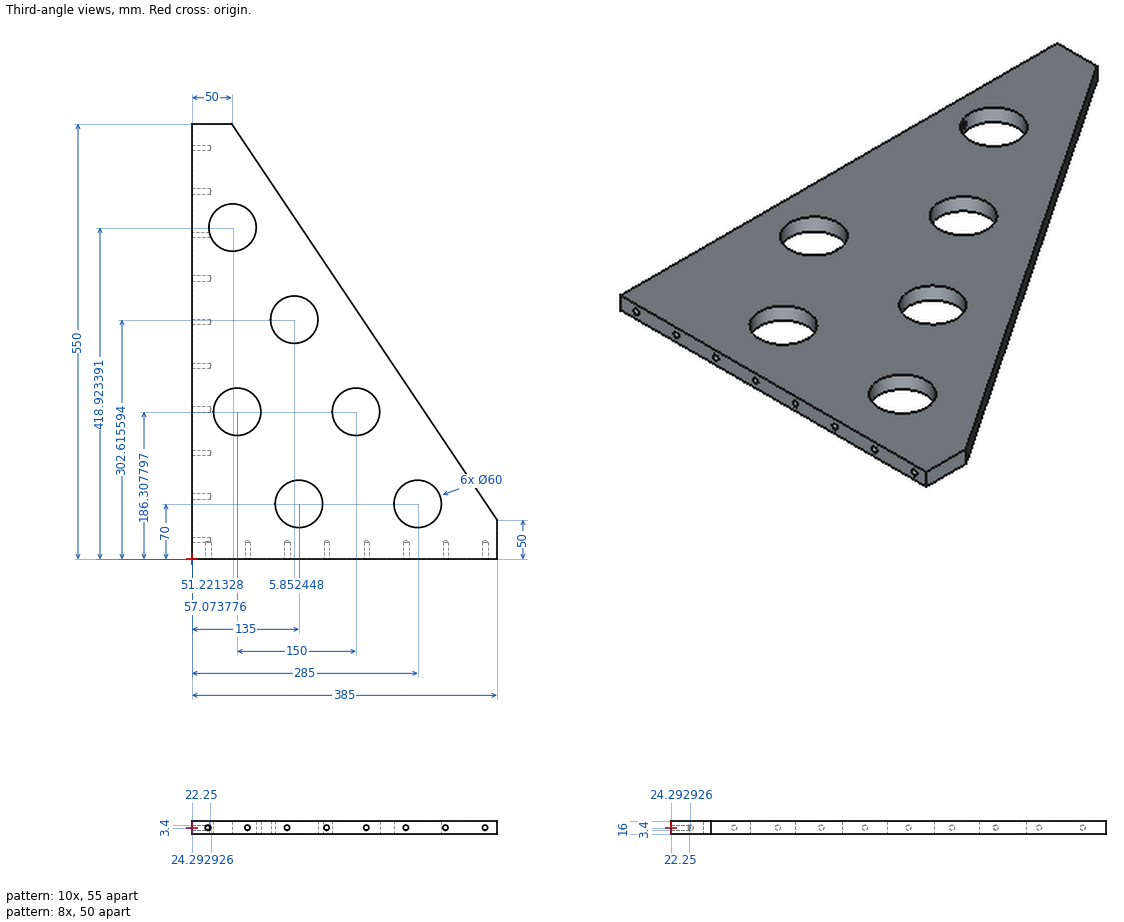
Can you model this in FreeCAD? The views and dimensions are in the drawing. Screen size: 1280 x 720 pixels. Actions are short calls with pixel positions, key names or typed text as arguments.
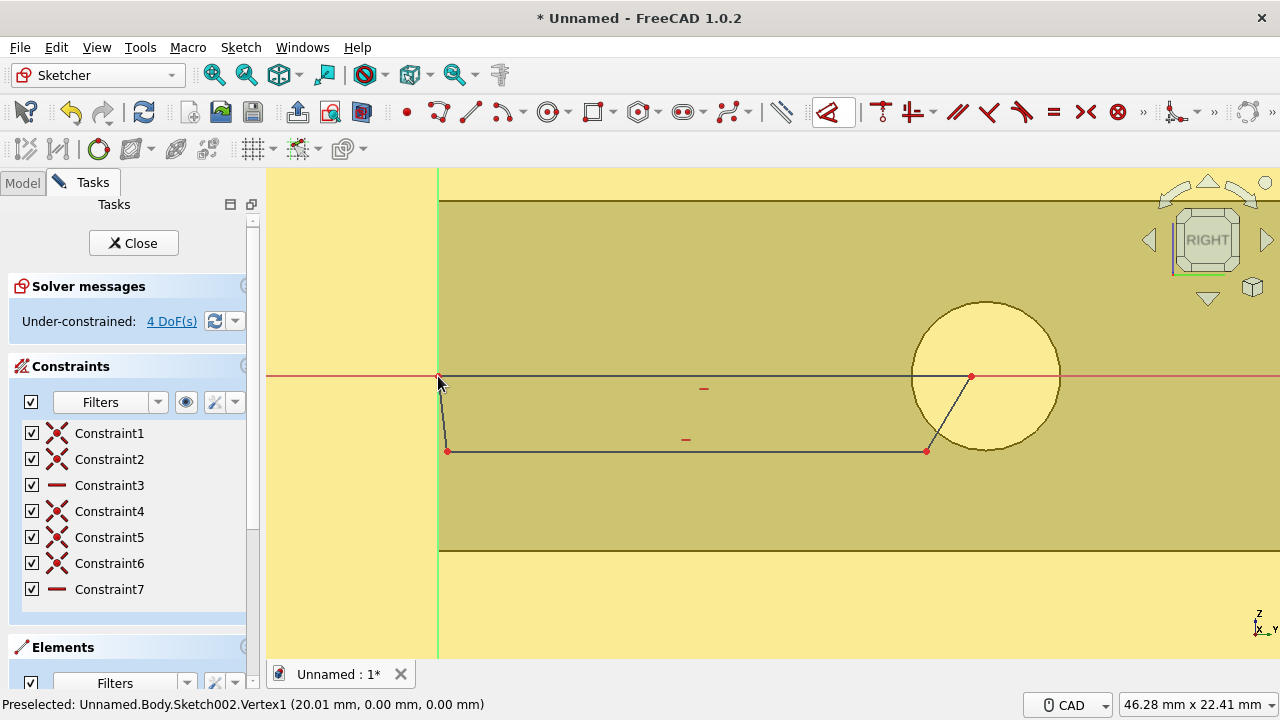
click(441, 399)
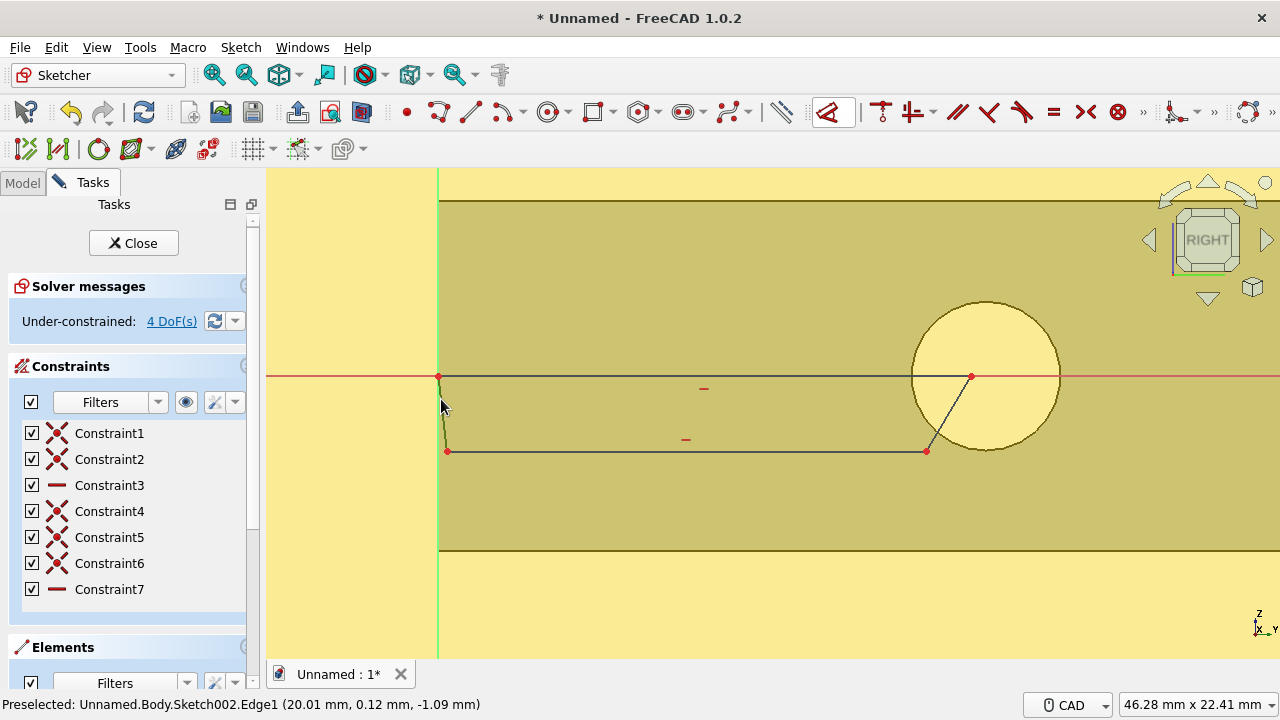
click(936, 112)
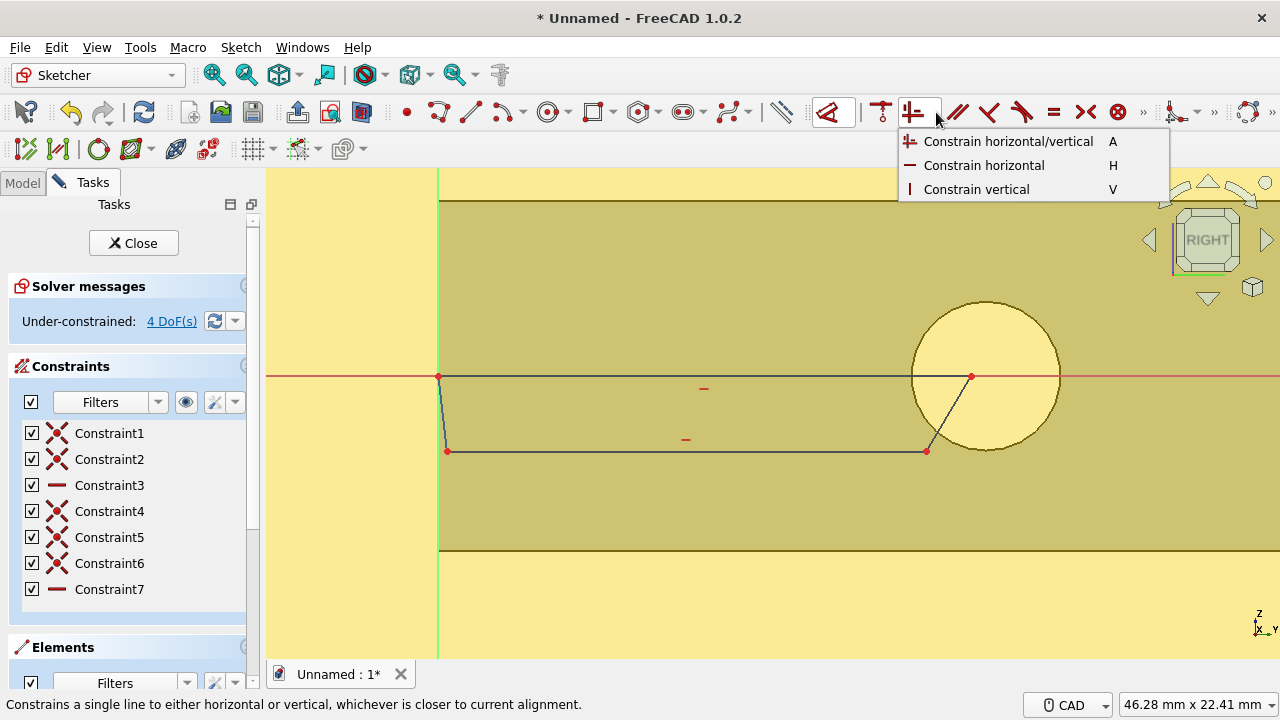
click(1034, 189)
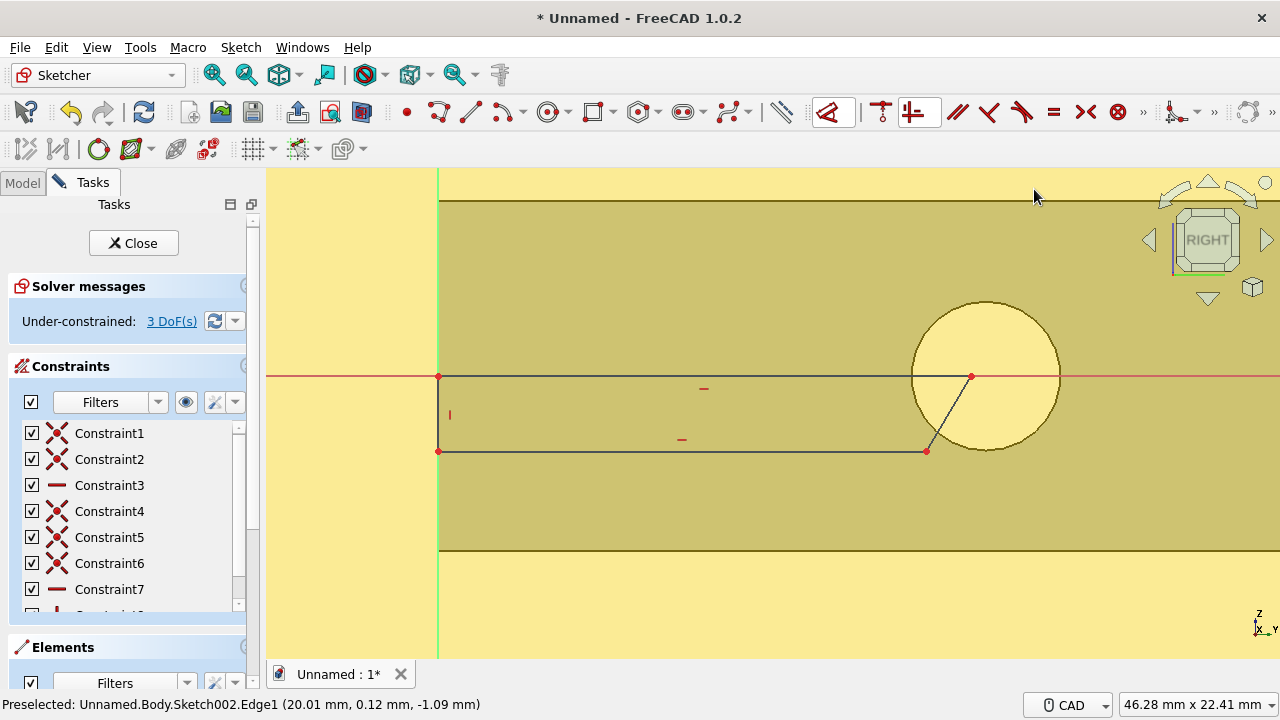
click(438, 399)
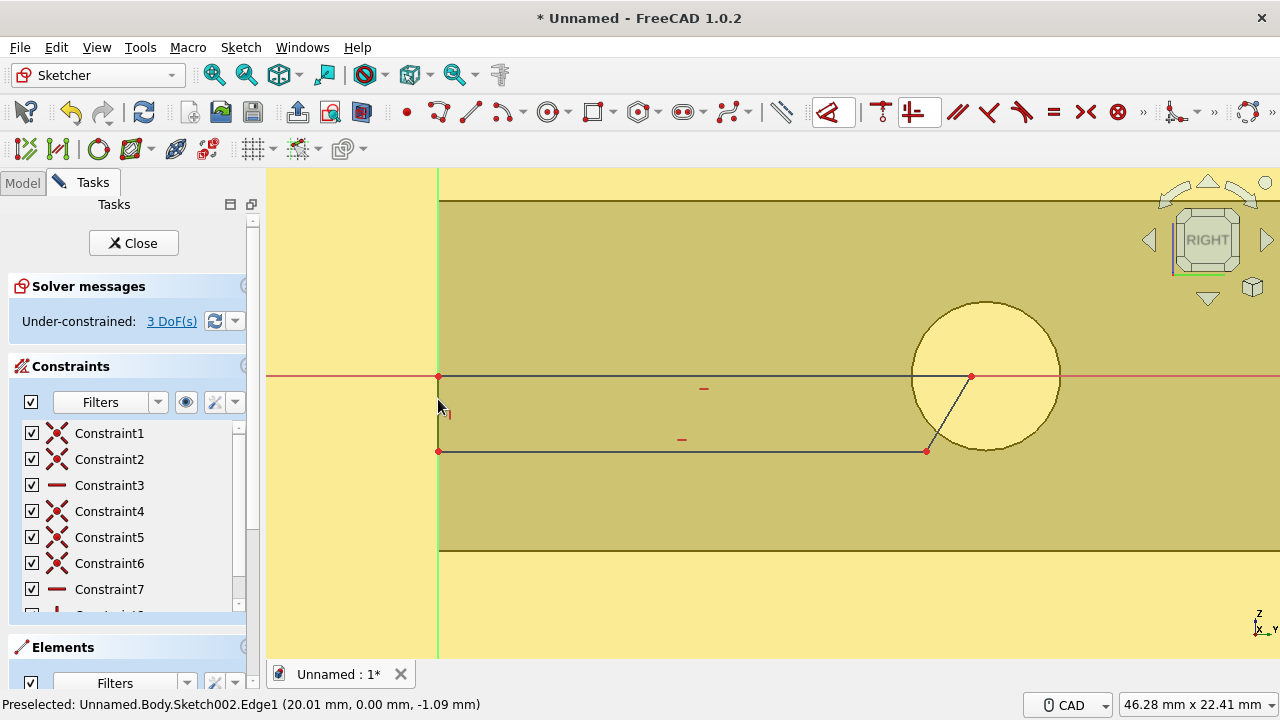
click(850, 112)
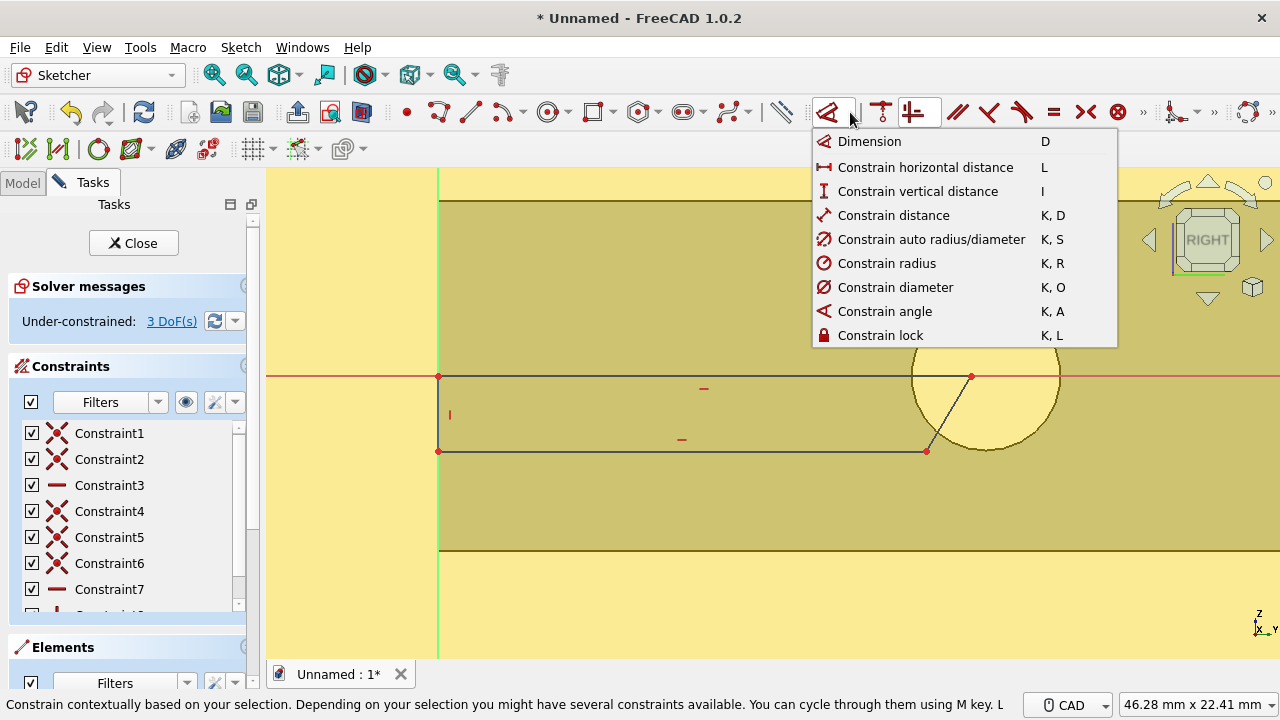
click(965, 191)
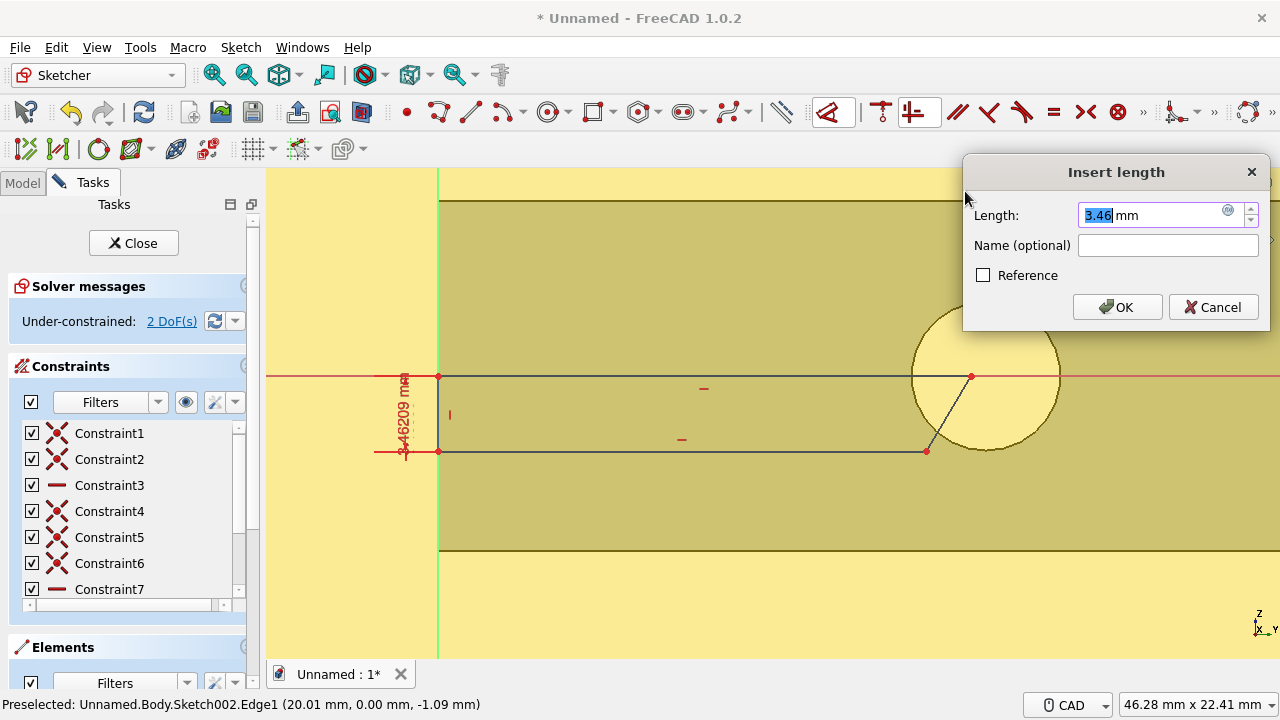
text(3.4)
key(Return)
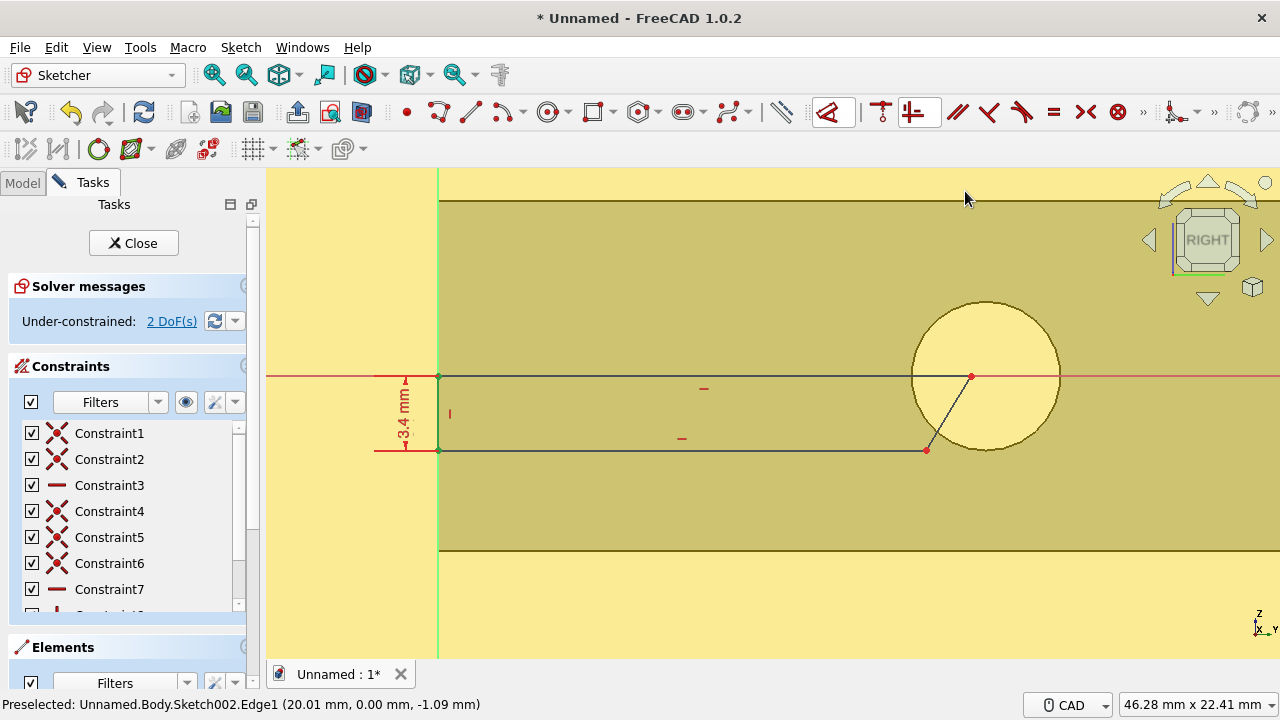
click(585, 451)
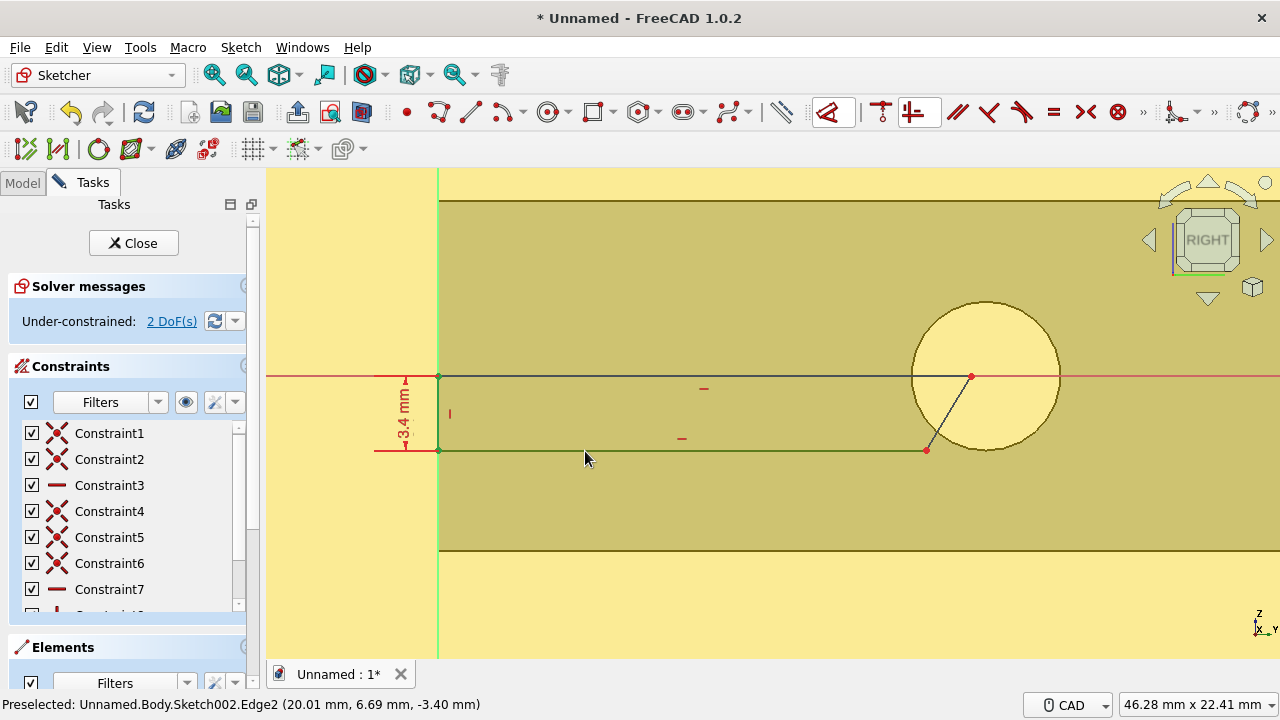
key(l)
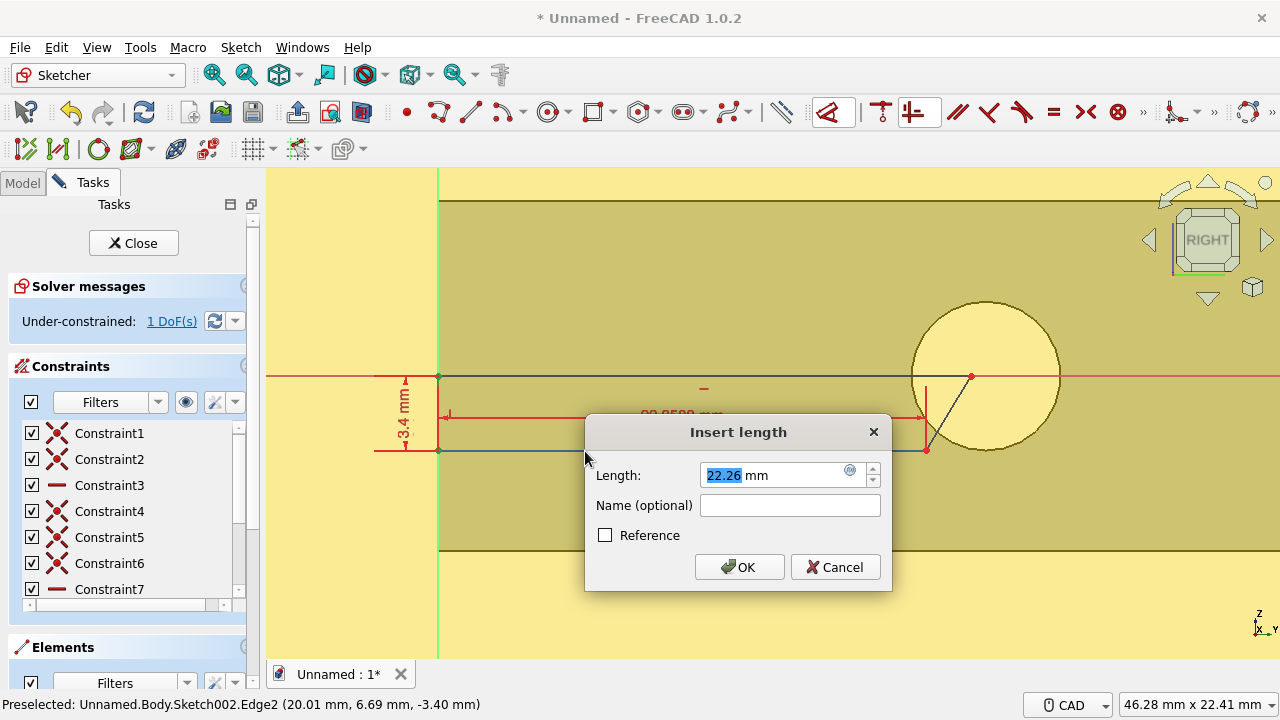
text(22.25)
key(Return)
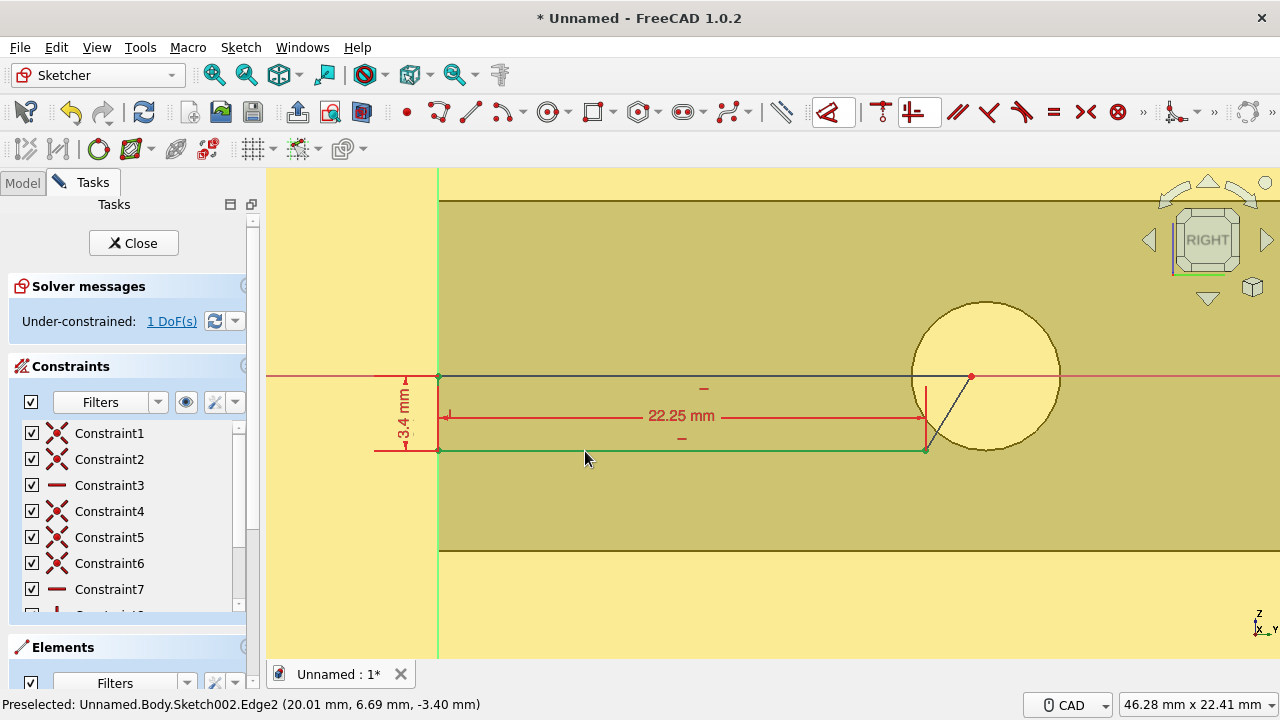
click(811, 376)